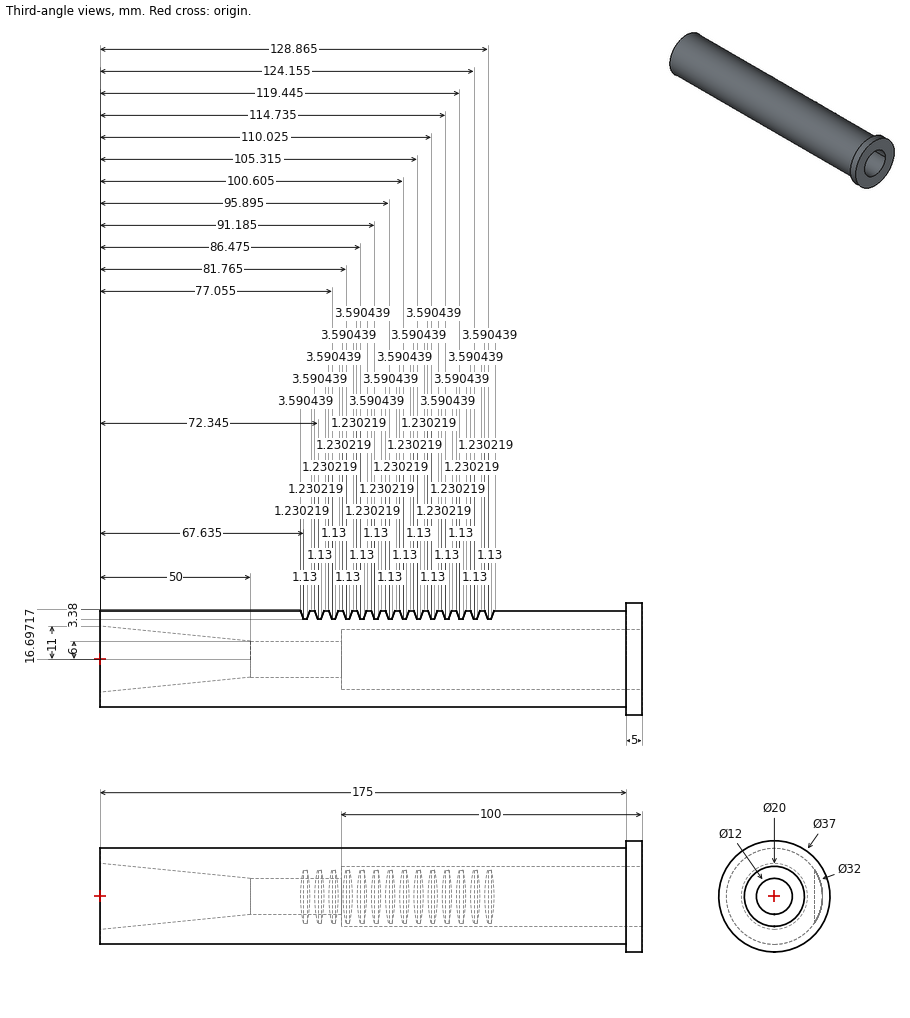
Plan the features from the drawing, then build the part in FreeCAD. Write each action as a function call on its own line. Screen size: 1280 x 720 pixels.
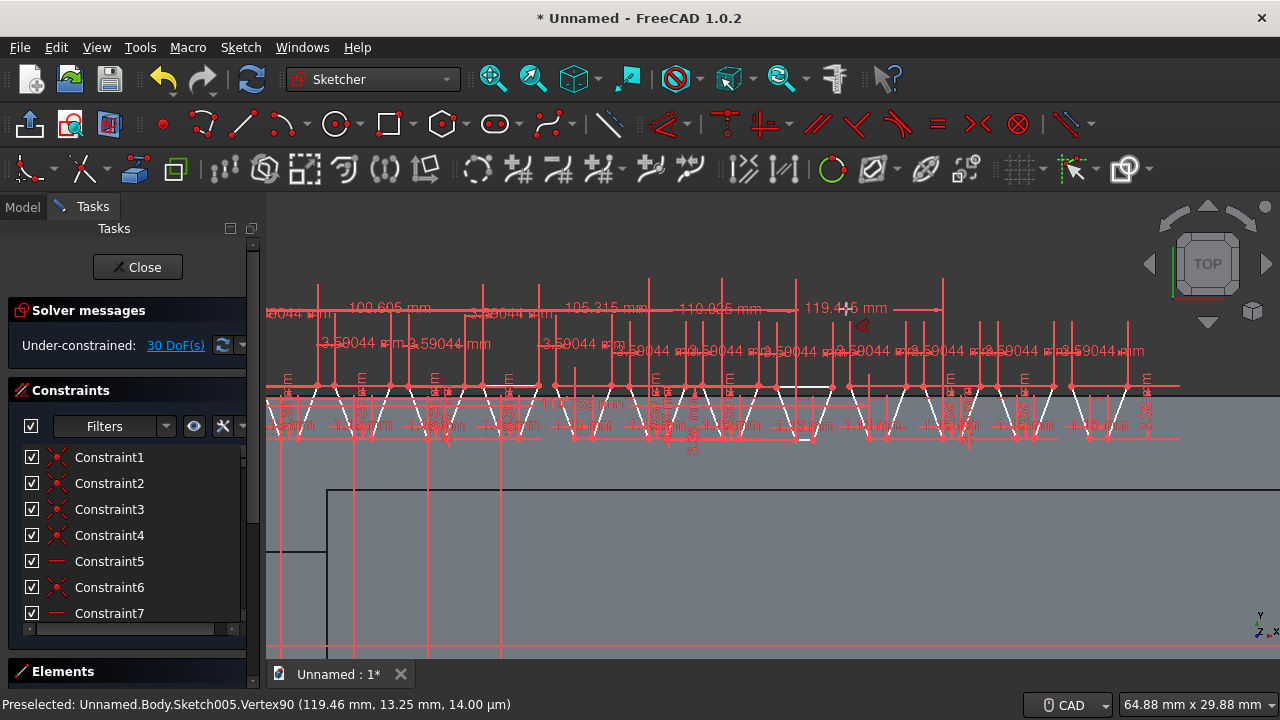
click(1017, 439)
click(655, 285)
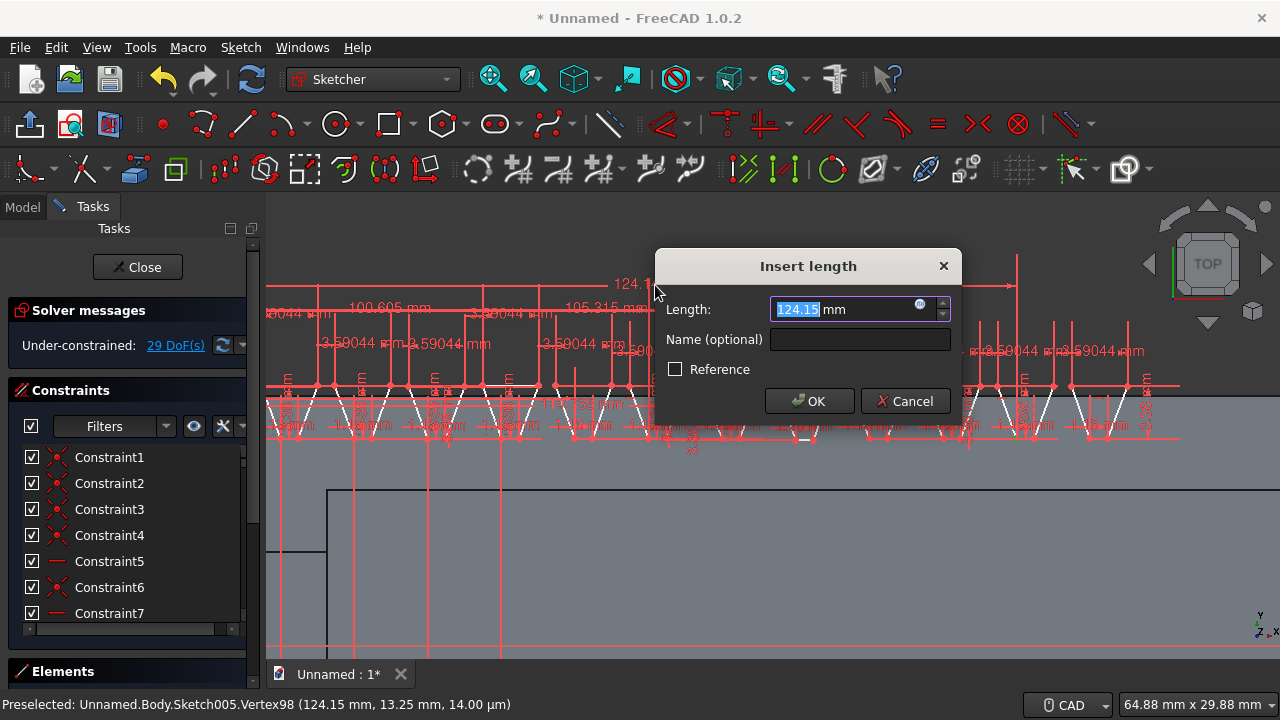
text(124.155)
key(Return)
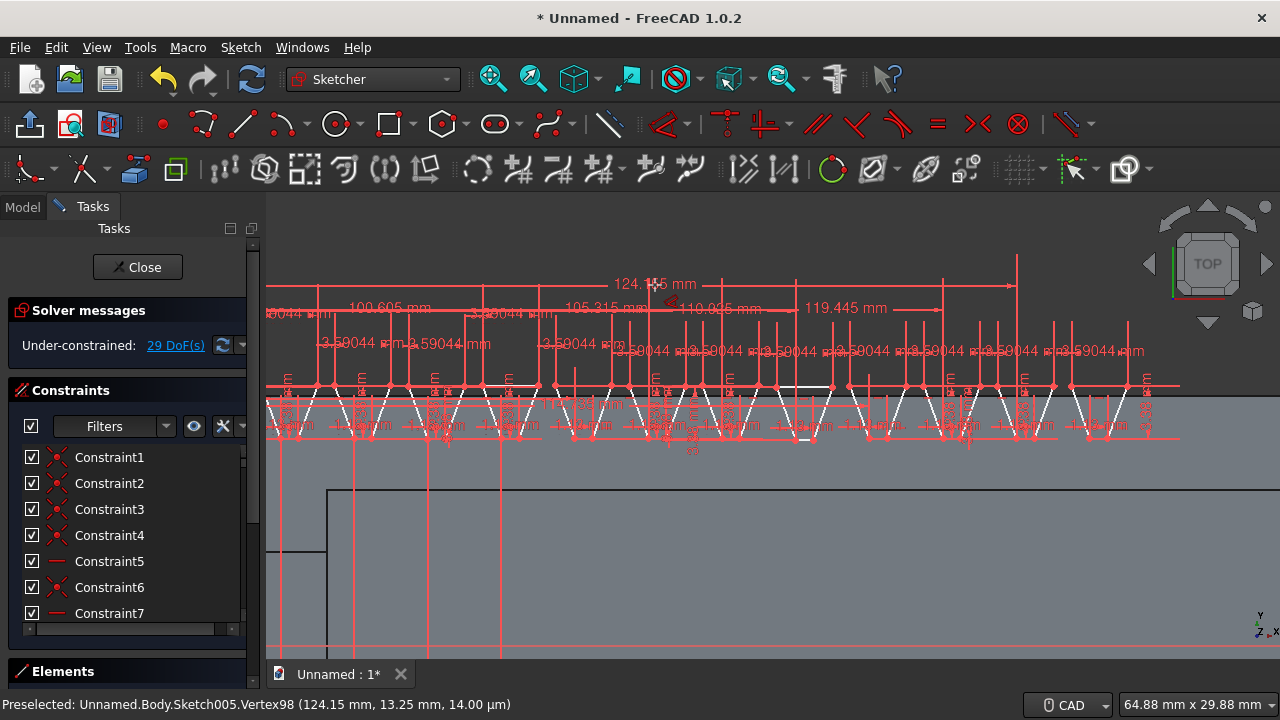
click(1090, 439)
click(875, 405)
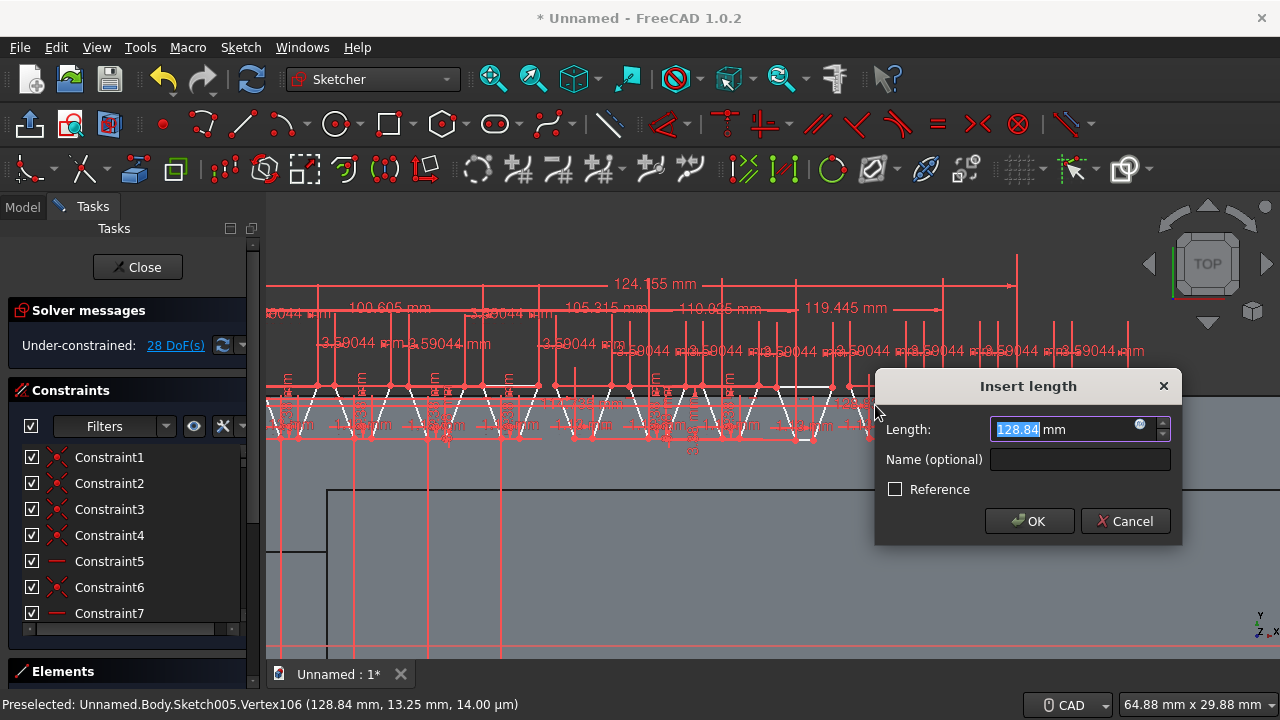
text(128.865)
key(Return)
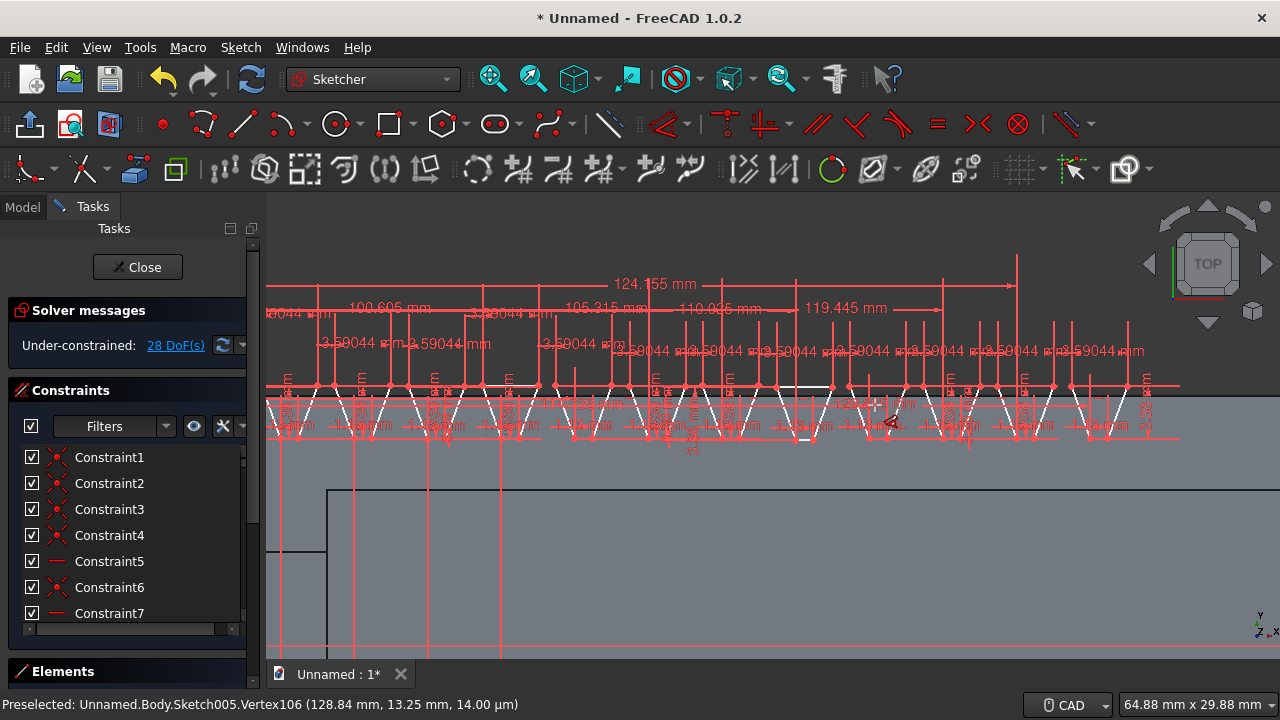
scroll(964, 387, down, 6)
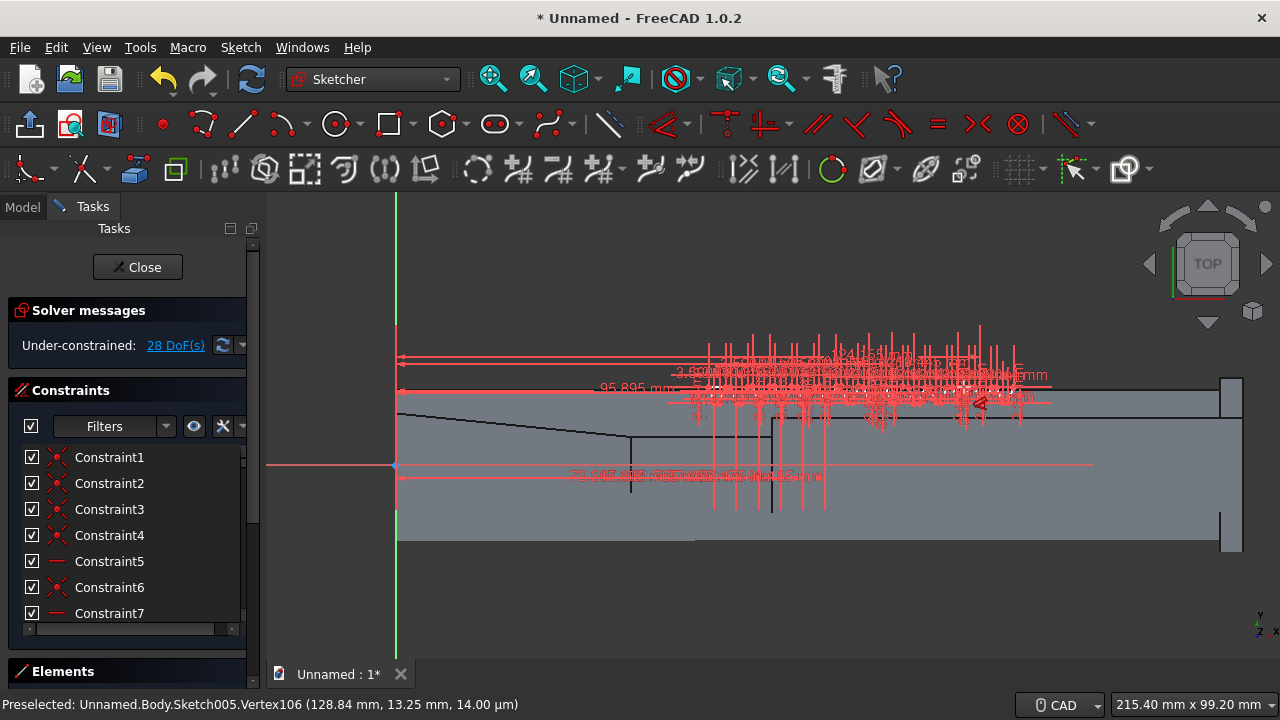
click(709, 387)
click(362, 426)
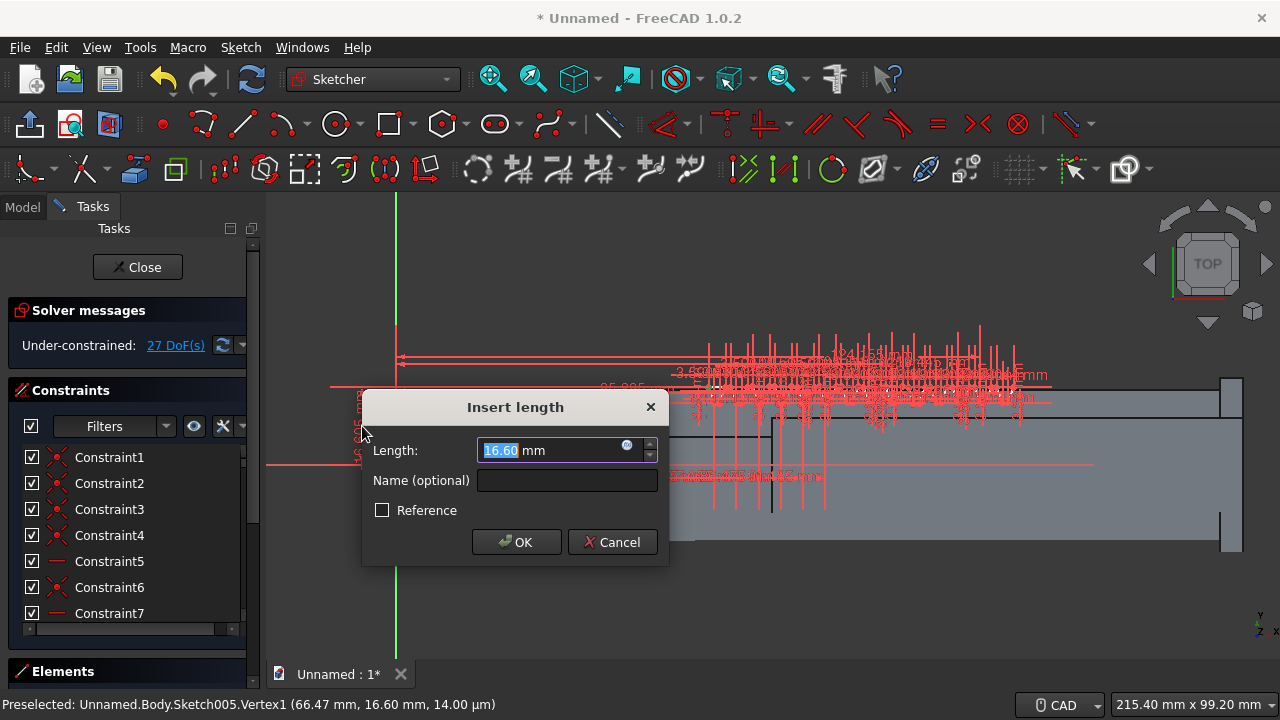
text(16.69717)
key(Return)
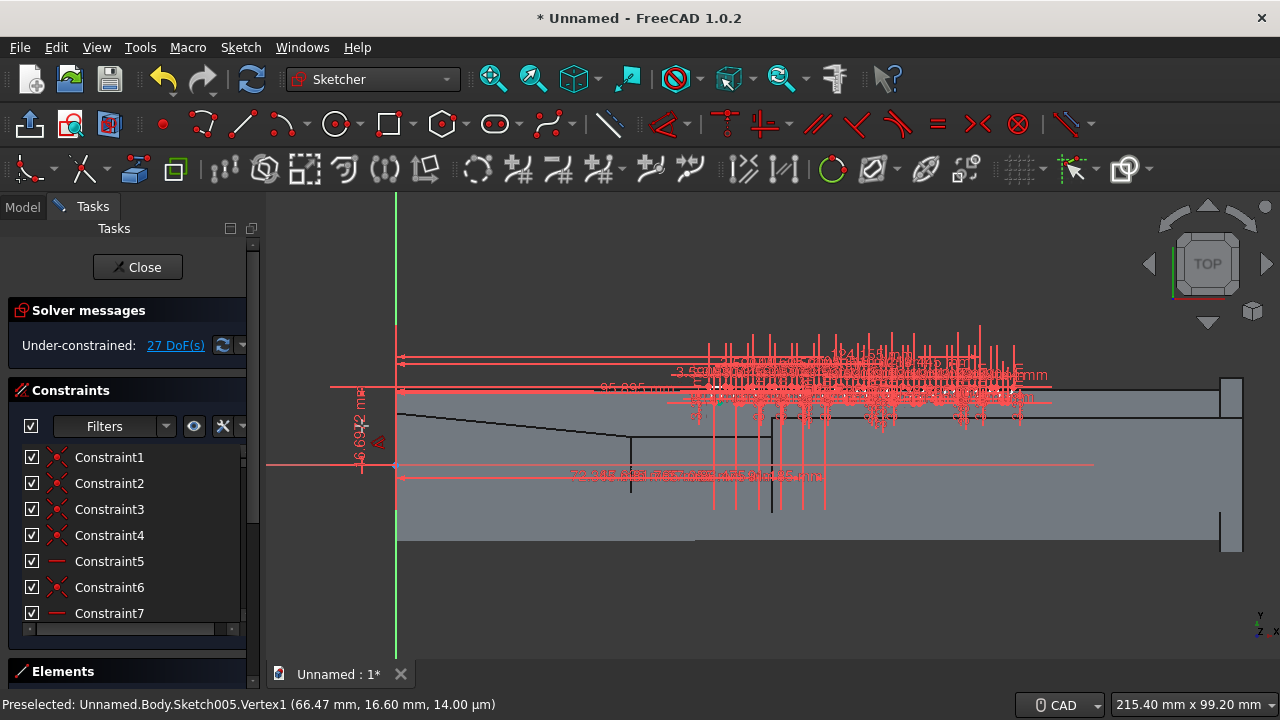
scroll(731, 387, up, 5)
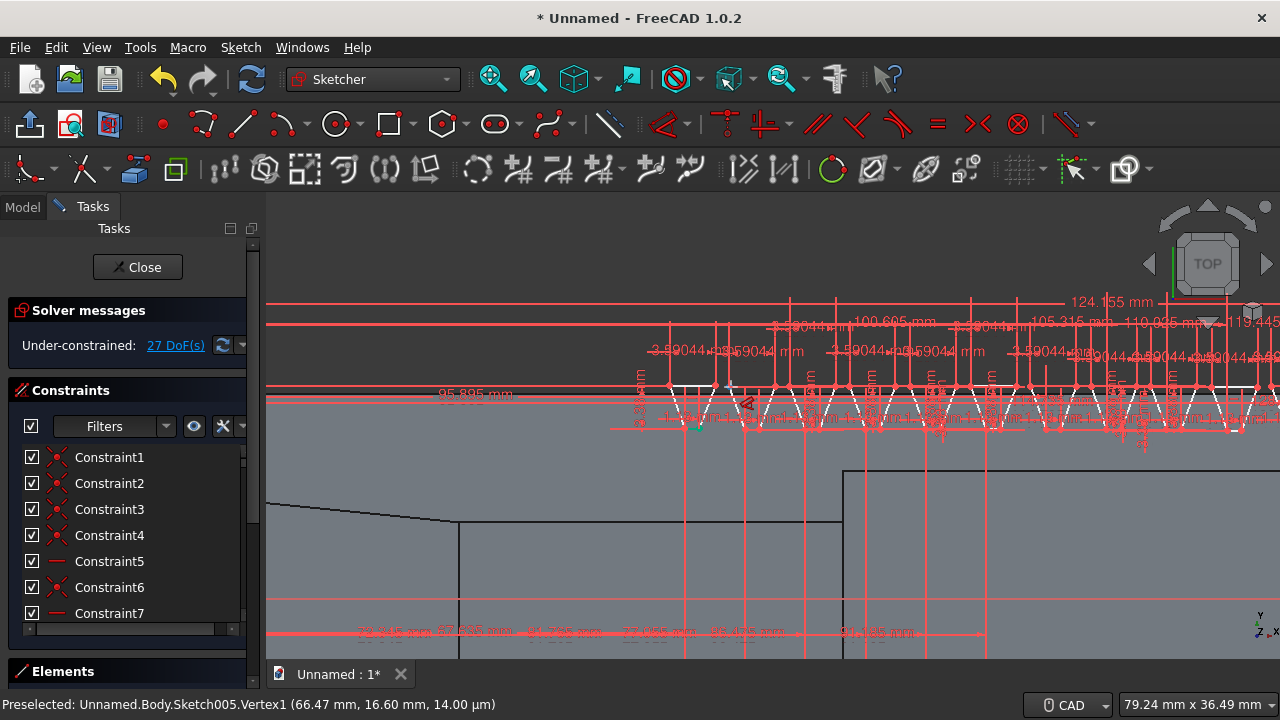
click(729, 387)
click(763, 493)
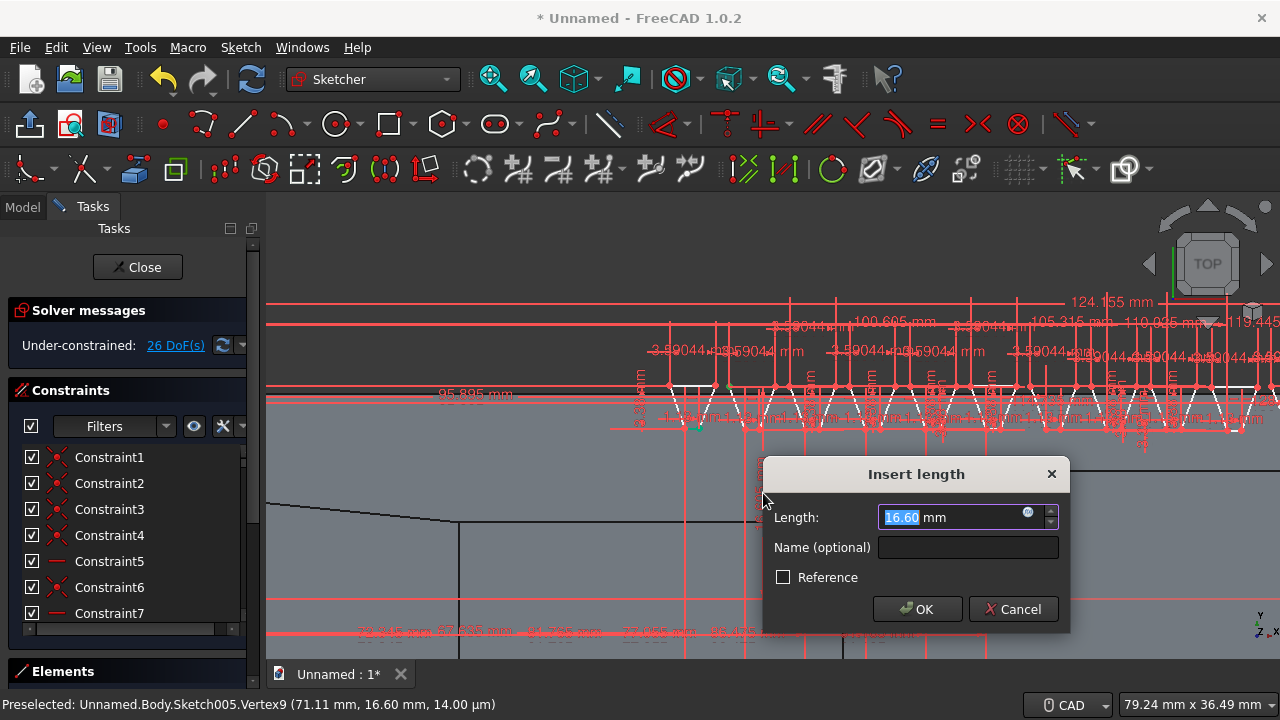
text(16.69717)
key(Return)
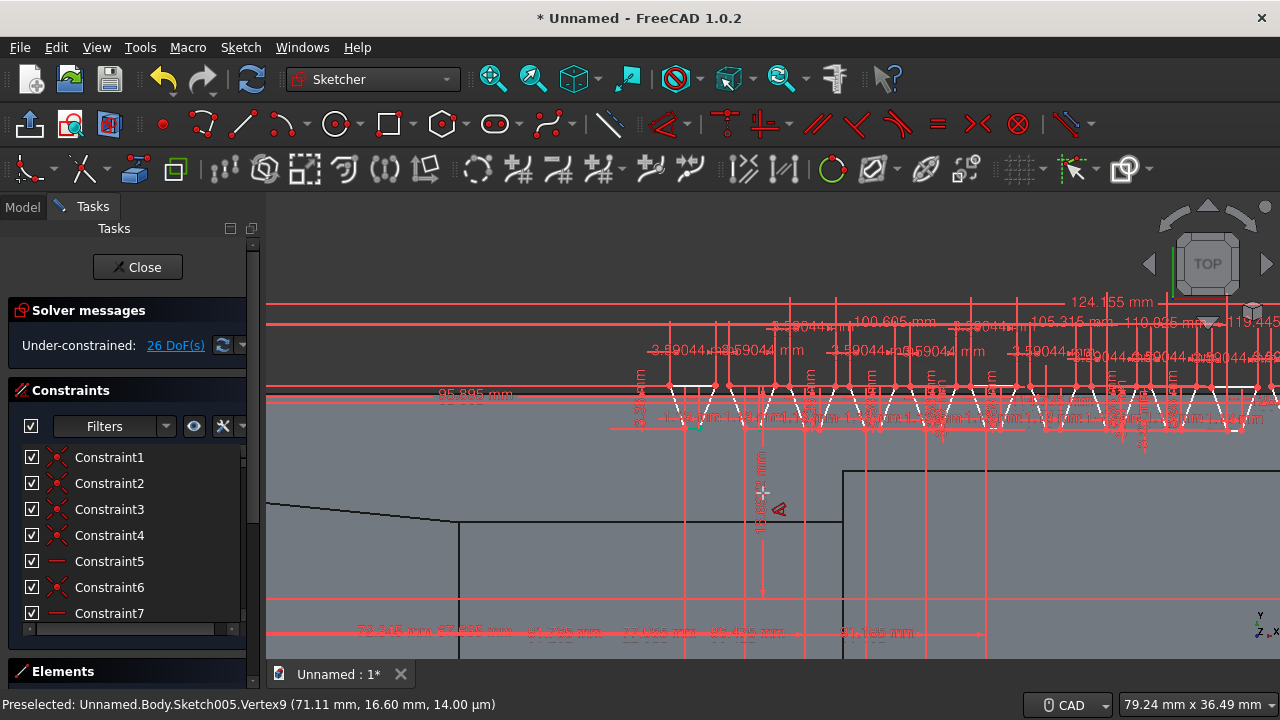
click(790, 386)
click(824, 444)